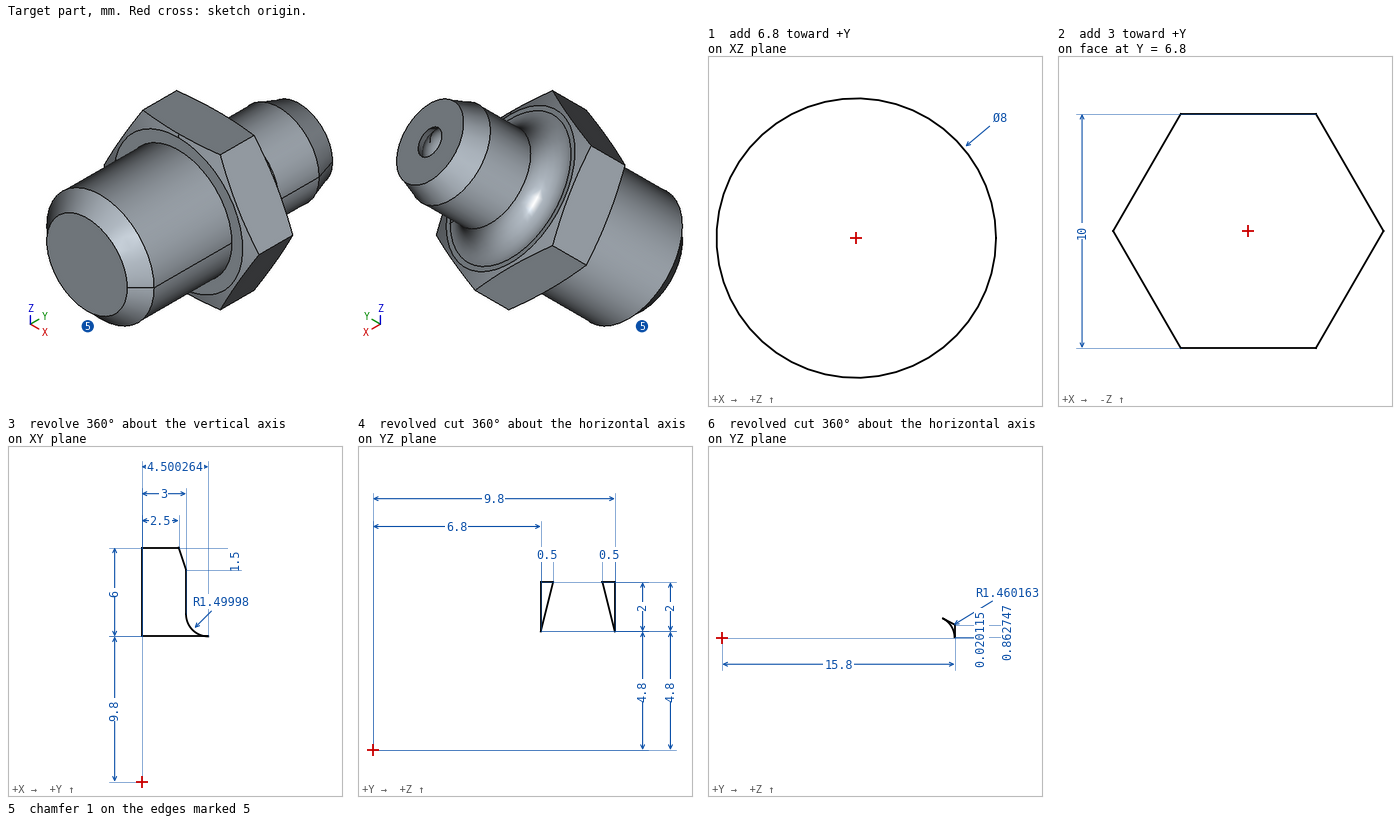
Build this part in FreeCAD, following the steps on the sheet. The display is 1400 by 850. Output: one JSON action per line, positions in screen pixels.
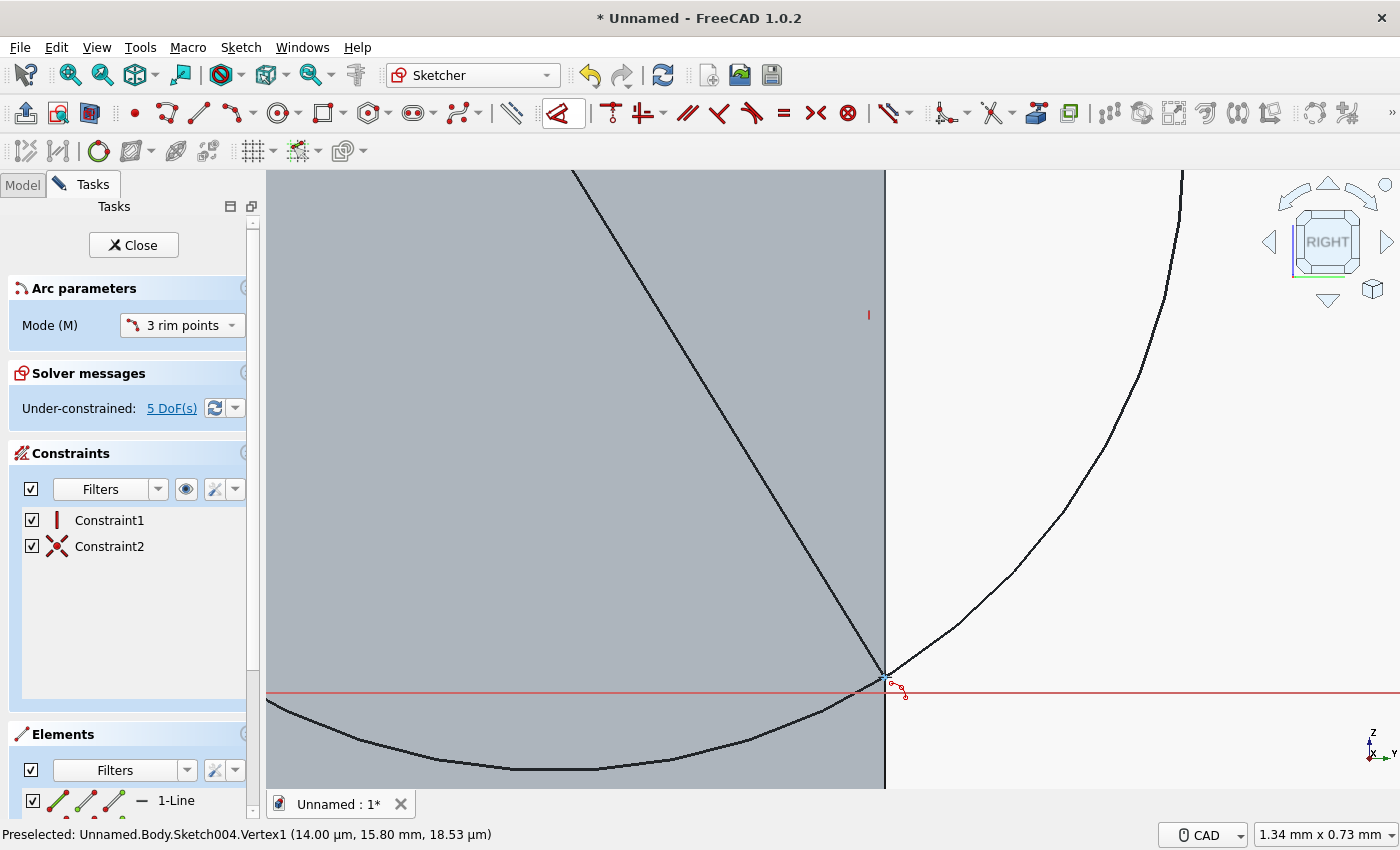
{"action": "scroll", "coordinate": [886, 678], "scroll_direction": "down", "scroll_amount": 5}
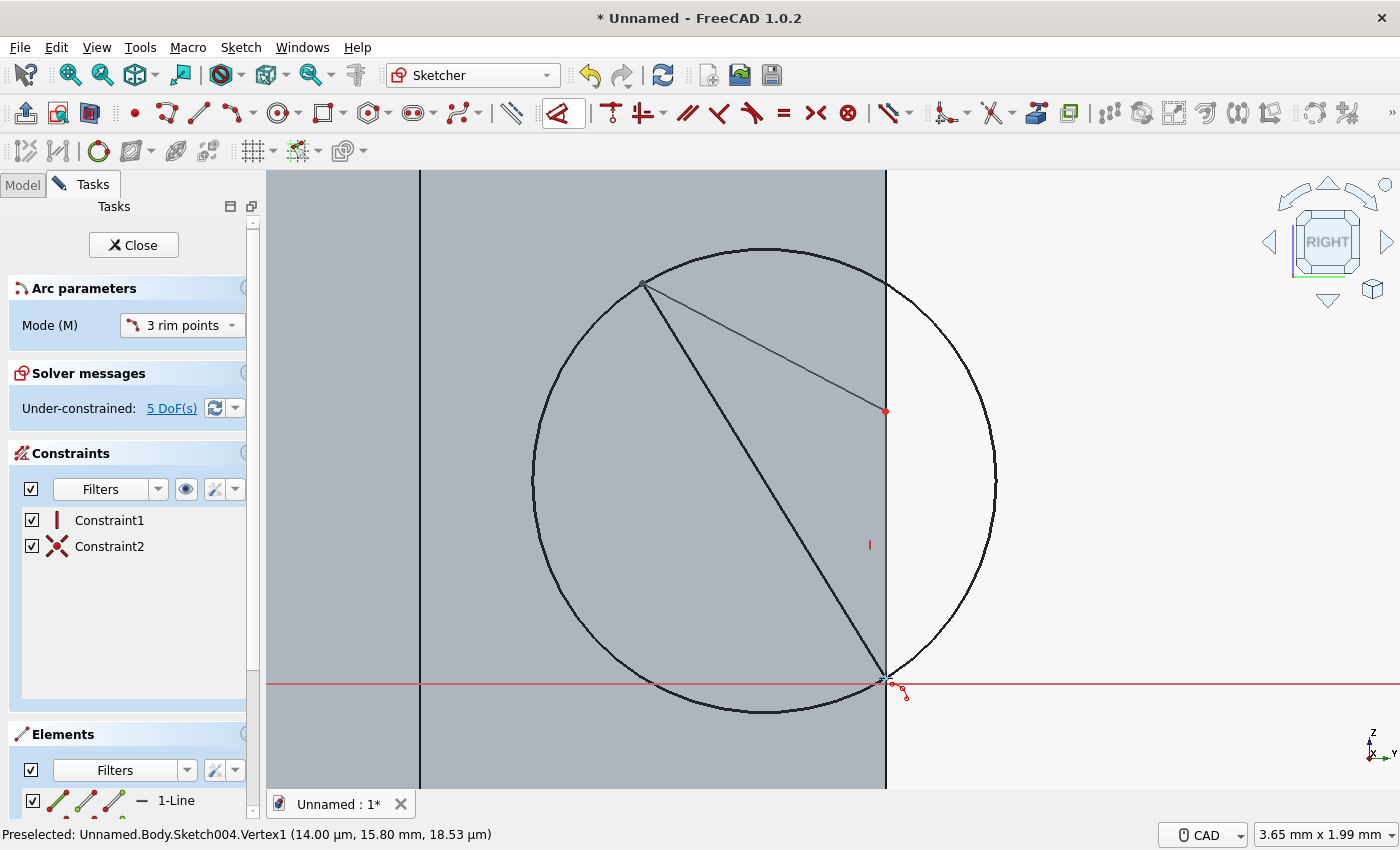
{"action": "left_click", "coordinate": [819, 447]}
{"action": "key", "text": "Escape"}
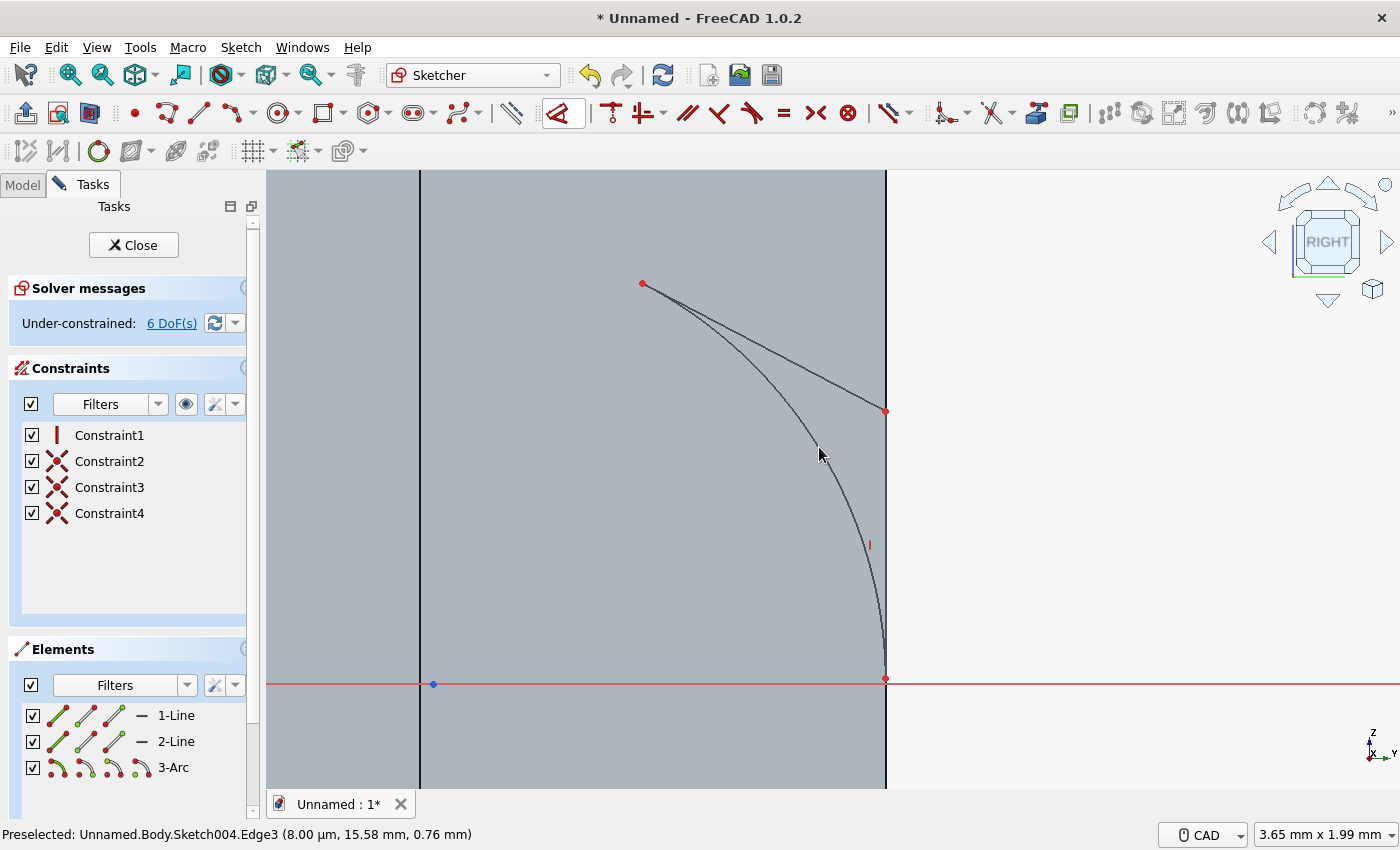
{"action": "left_click", "coordinate": [813, 373]}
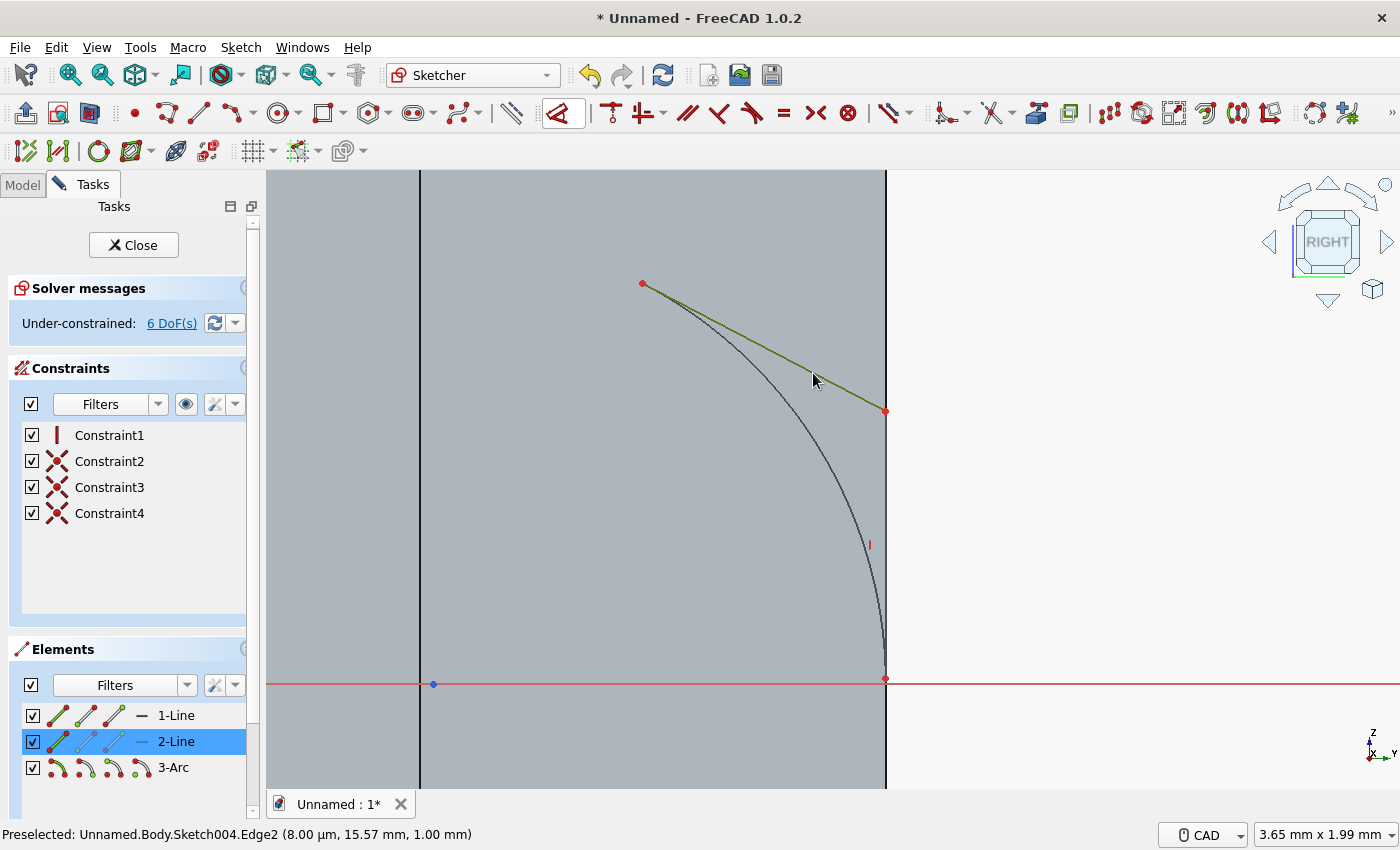
{"action": "left_click", "coordinate": [860, 535]}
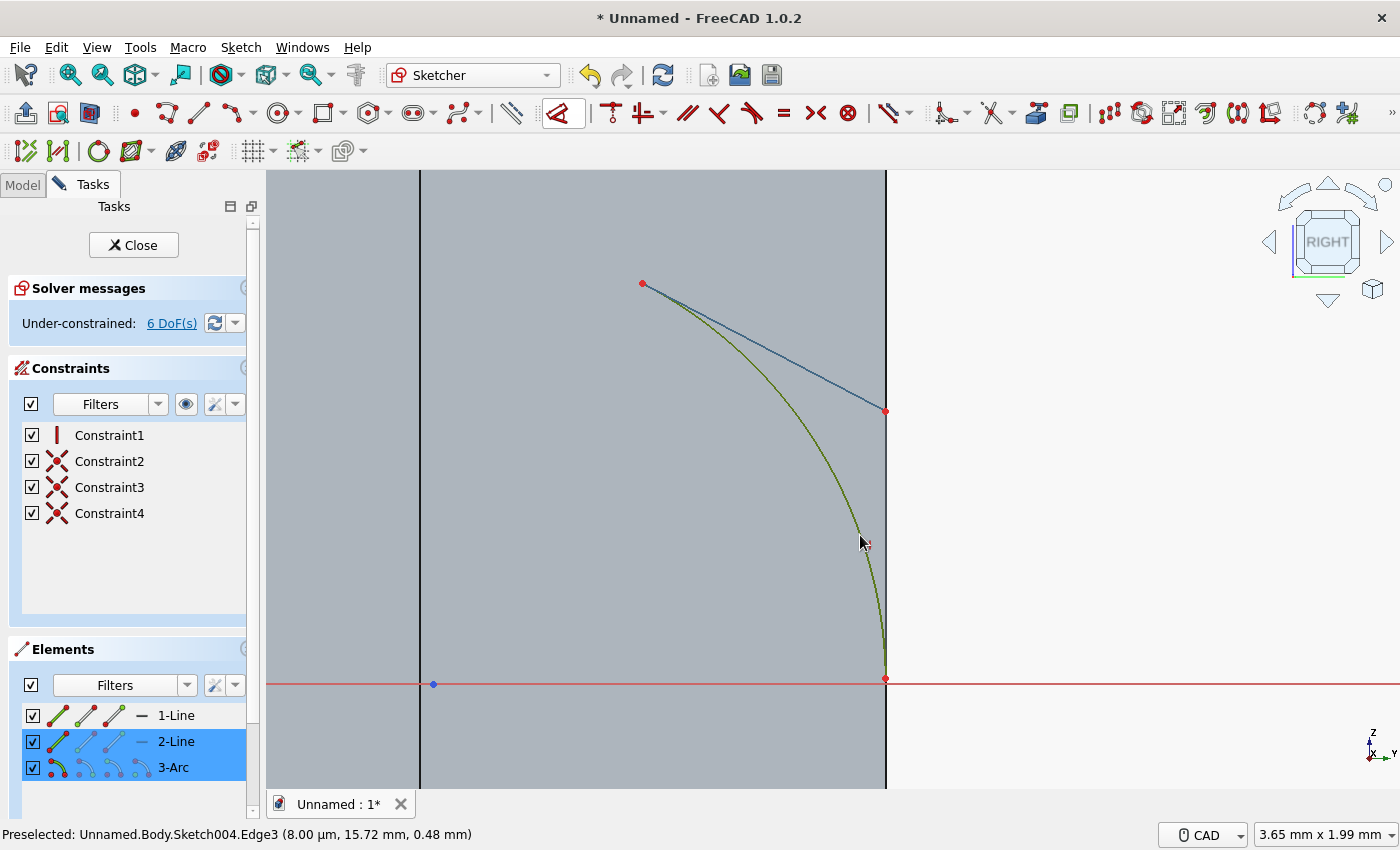
{"action": "key", "text": "t"}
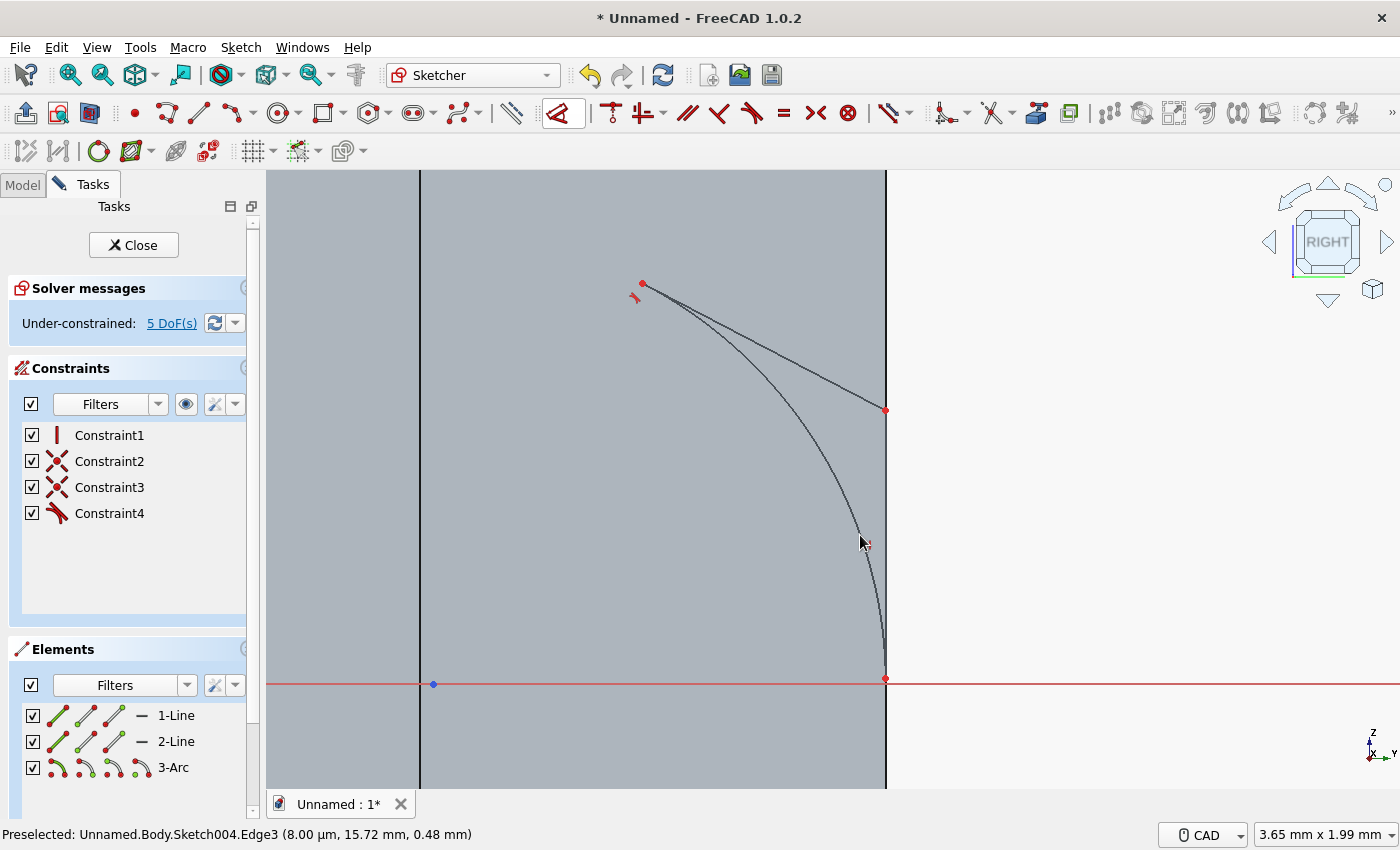
{"action": "left_click", "coordinate": [433, 685]}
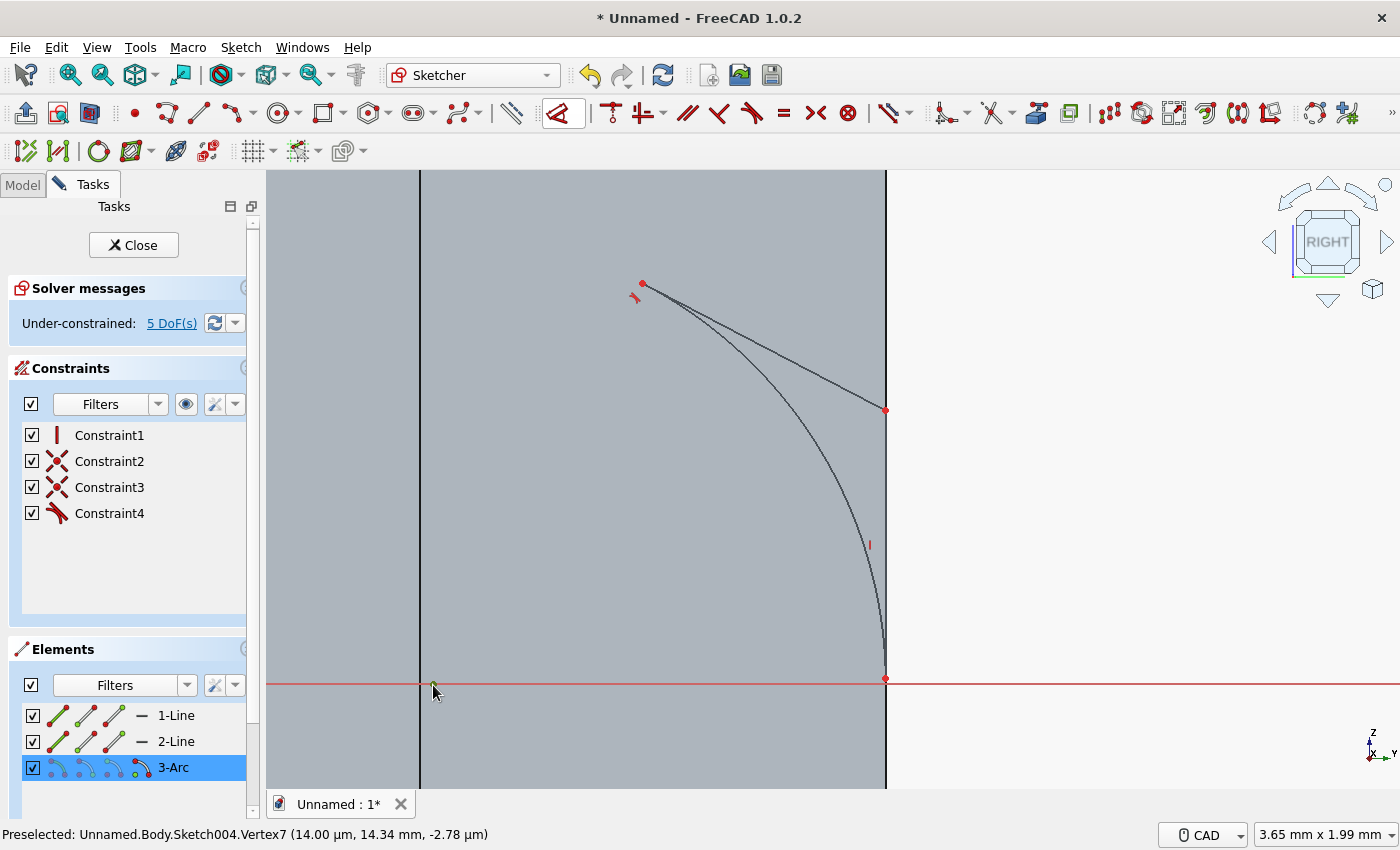
{"action": "left_click", "coordinate": [361, 684]}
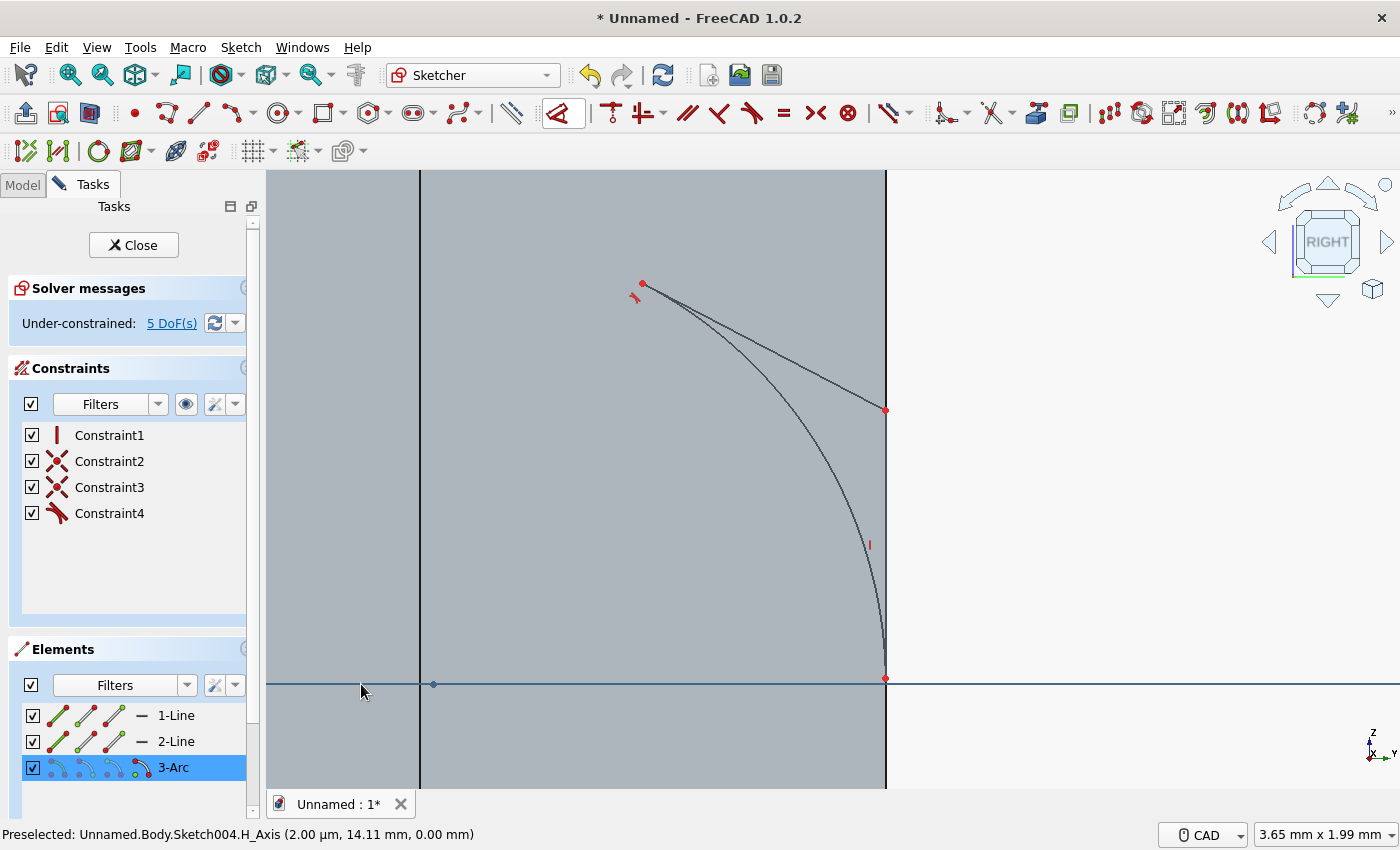
{"action": "left_click", "coordinate": [612, 114]}